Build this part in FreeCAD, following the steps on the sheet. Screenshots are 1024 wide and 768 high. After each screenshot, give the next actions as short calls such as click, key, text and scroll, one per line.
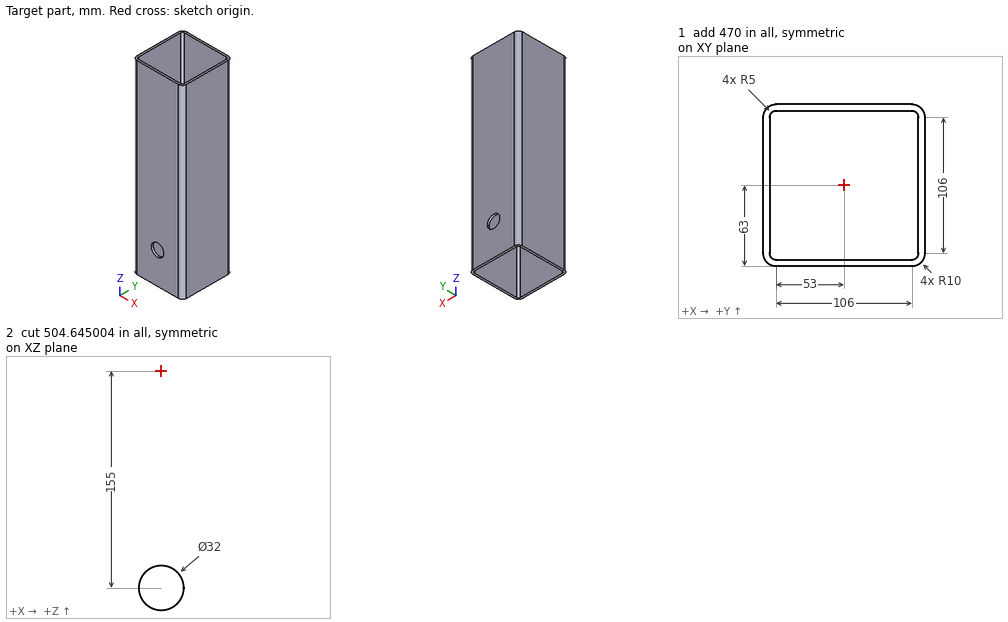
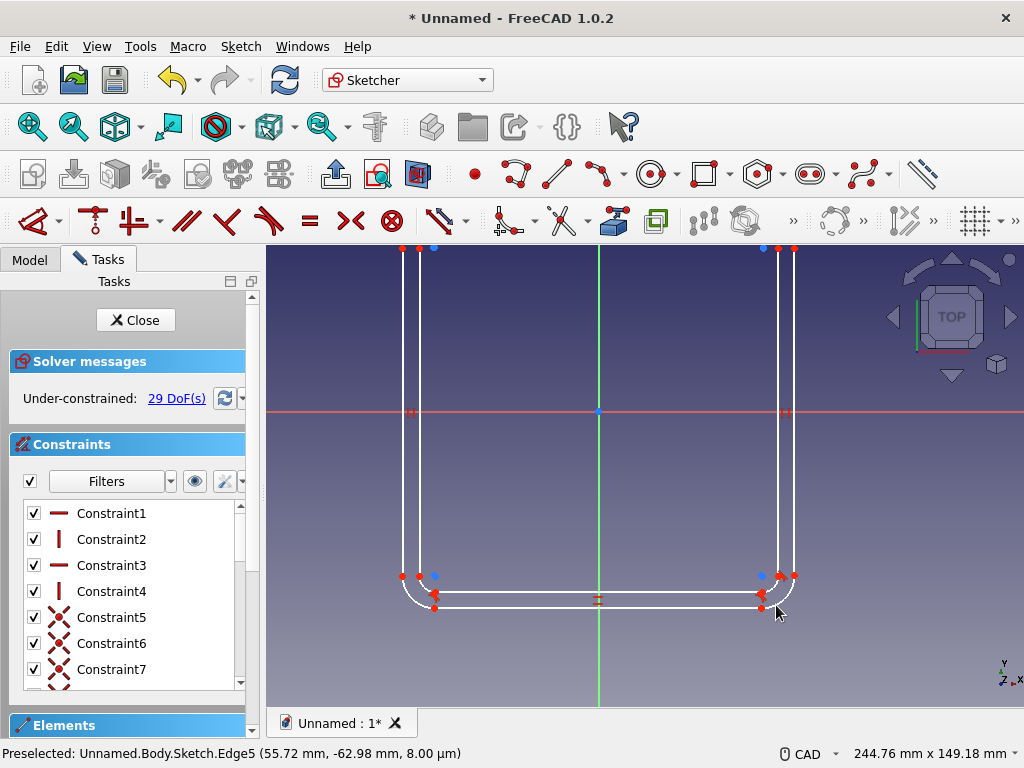
click(794, 477)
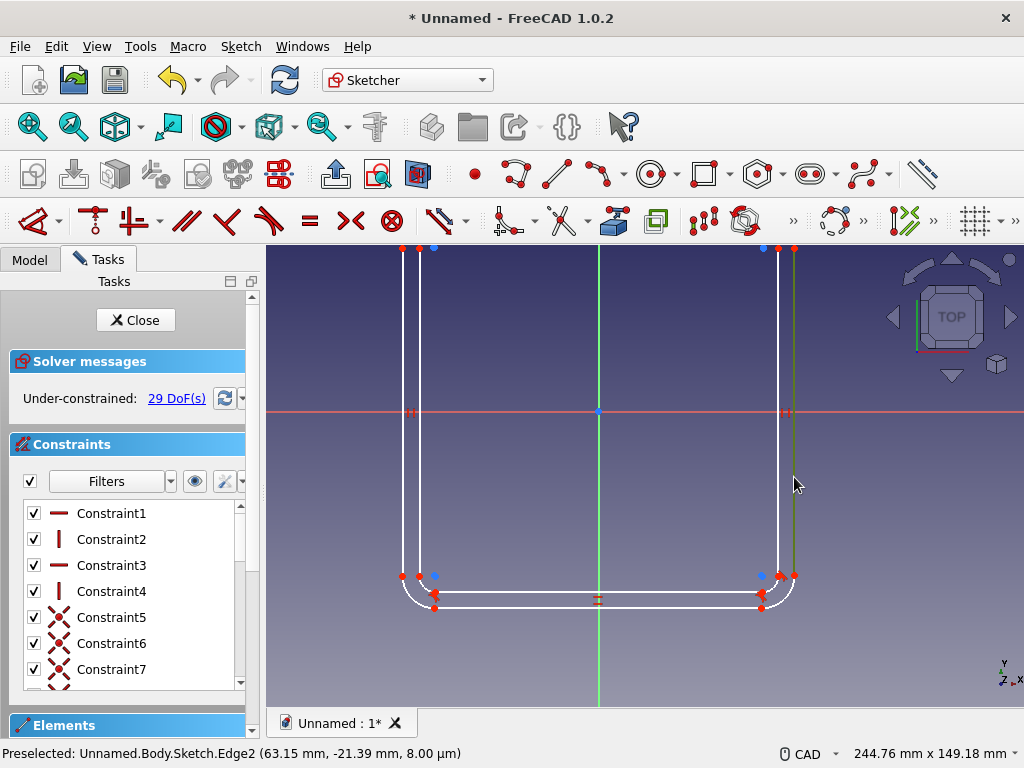
scroll(531, 607, down, 2)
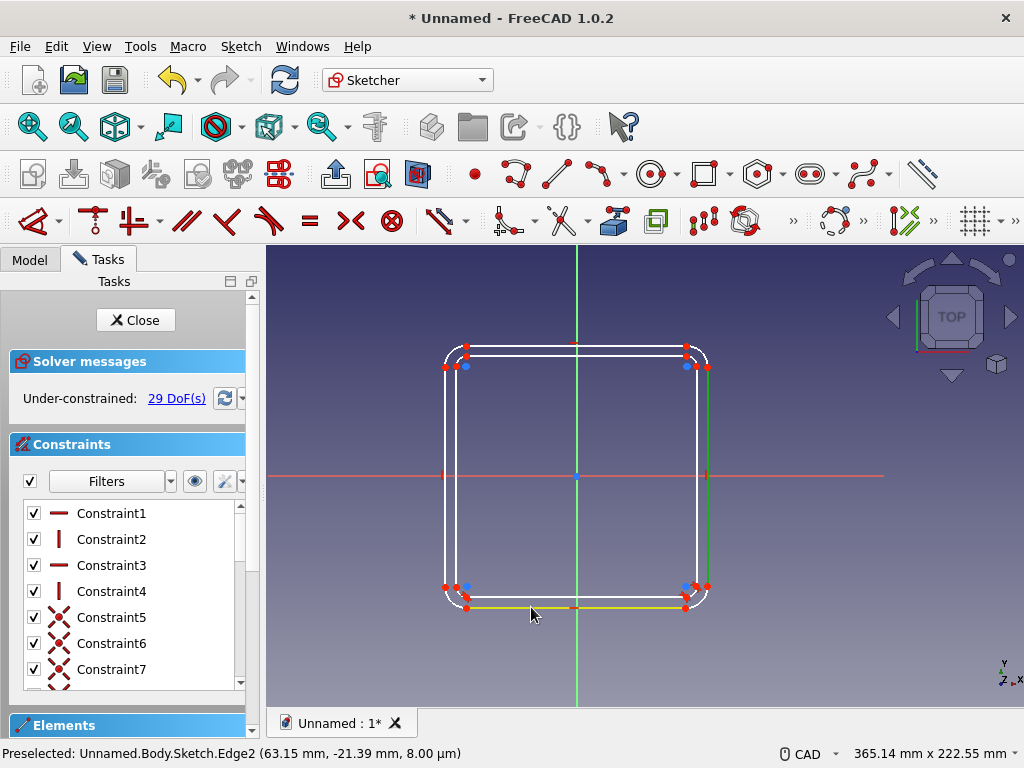
scroll(706, 358, up, 2)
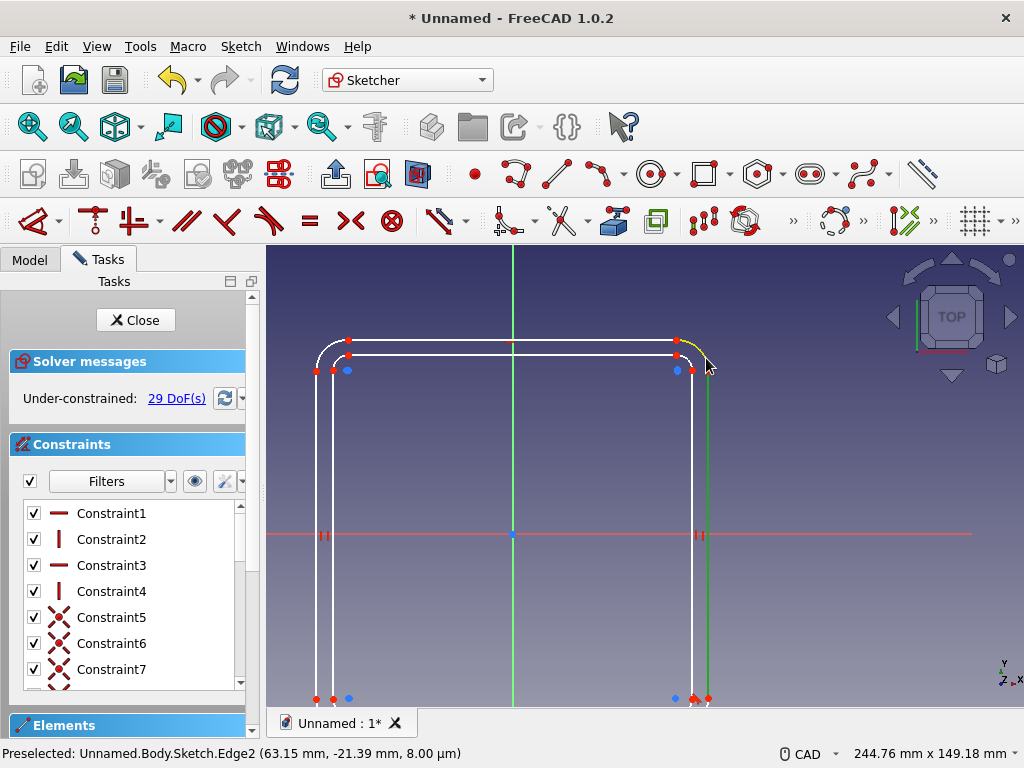
click(705, 357)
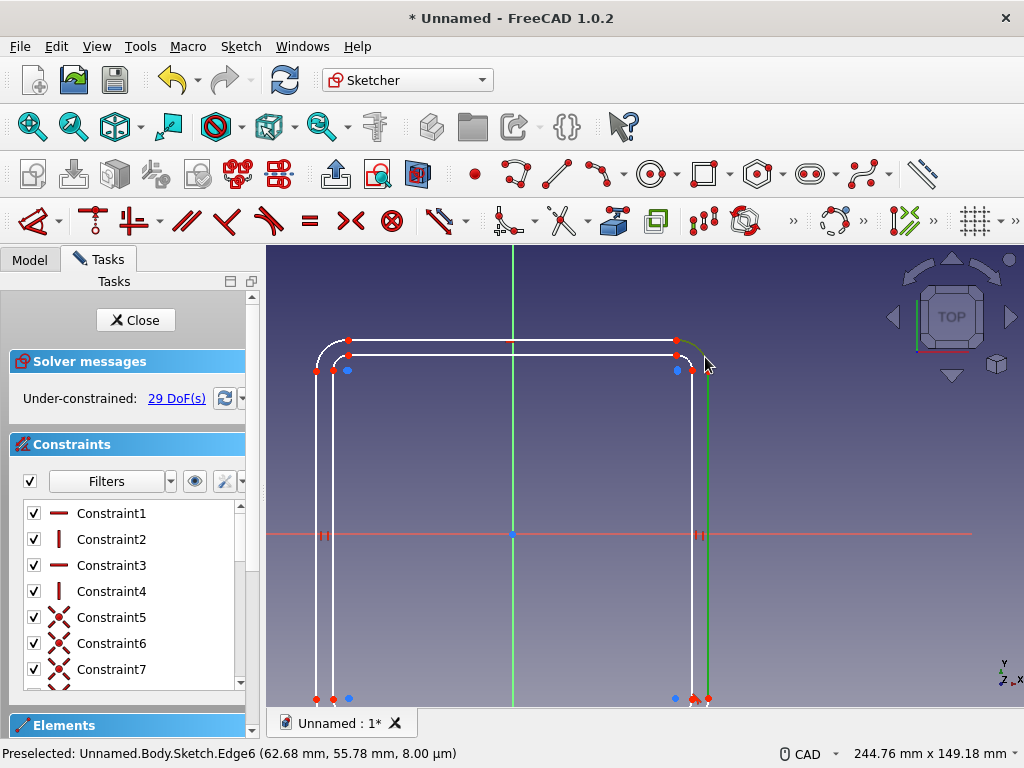
click(269, 222)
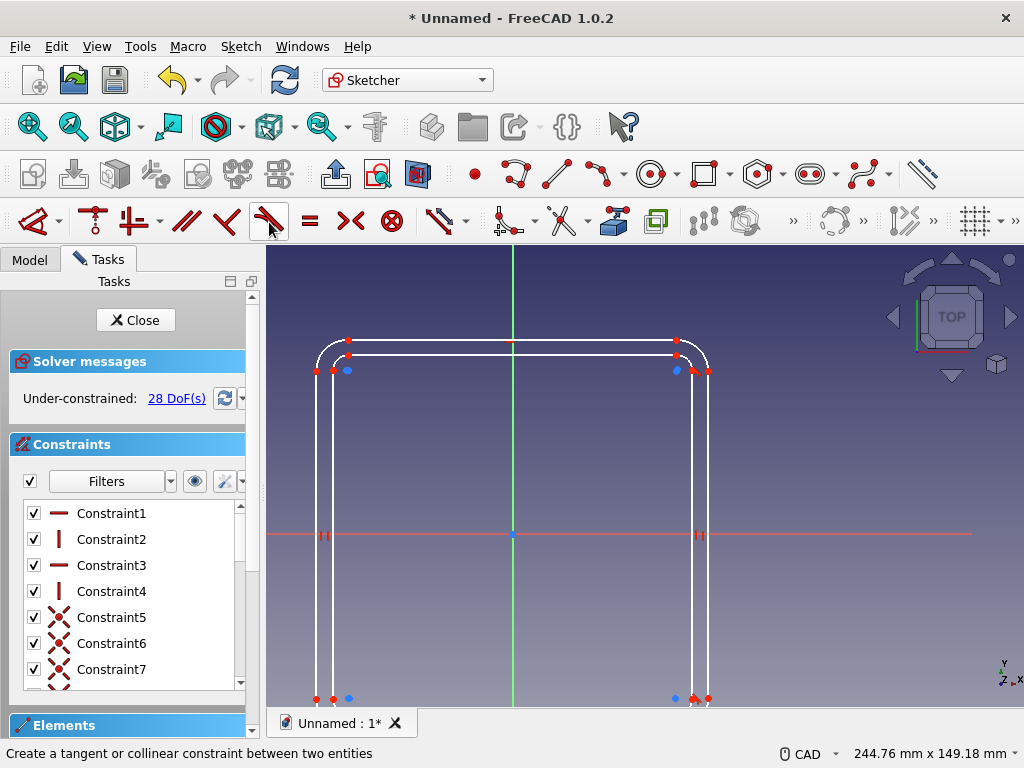
click(578, 340)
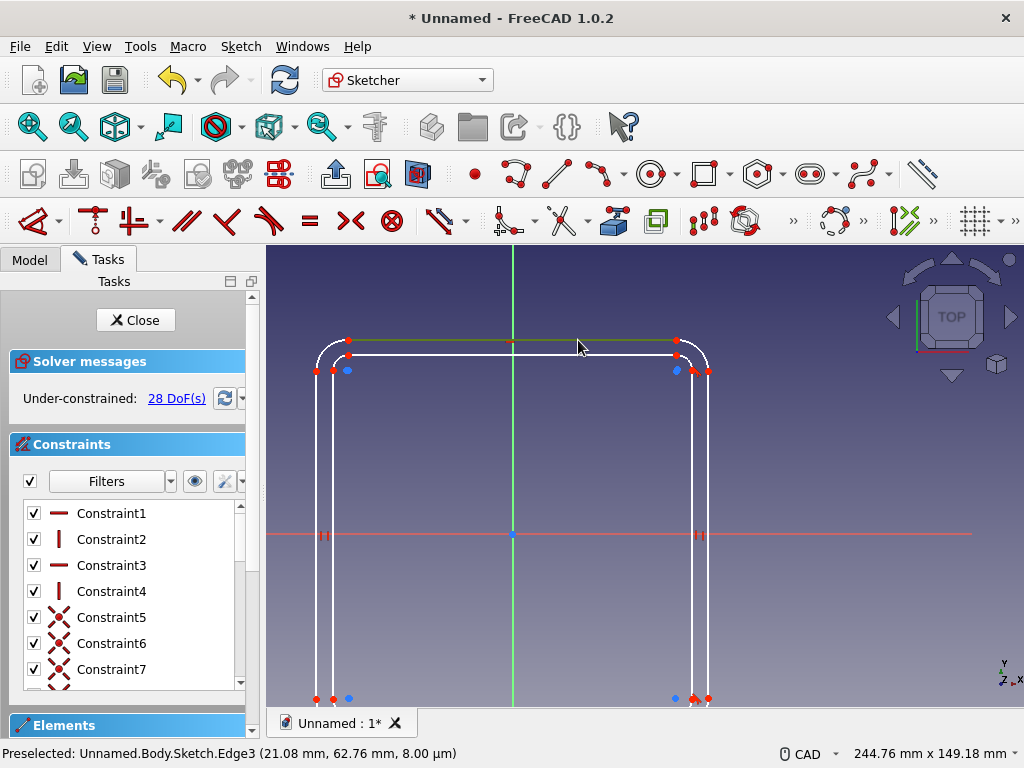
click(705, 357)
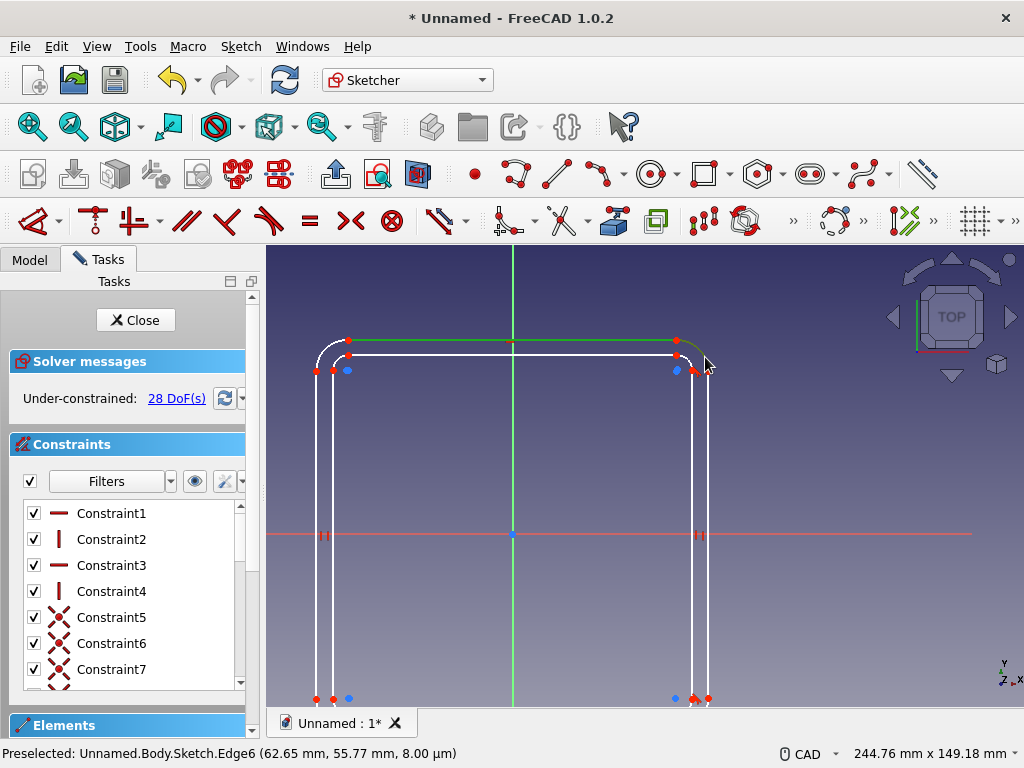
click(269, 222)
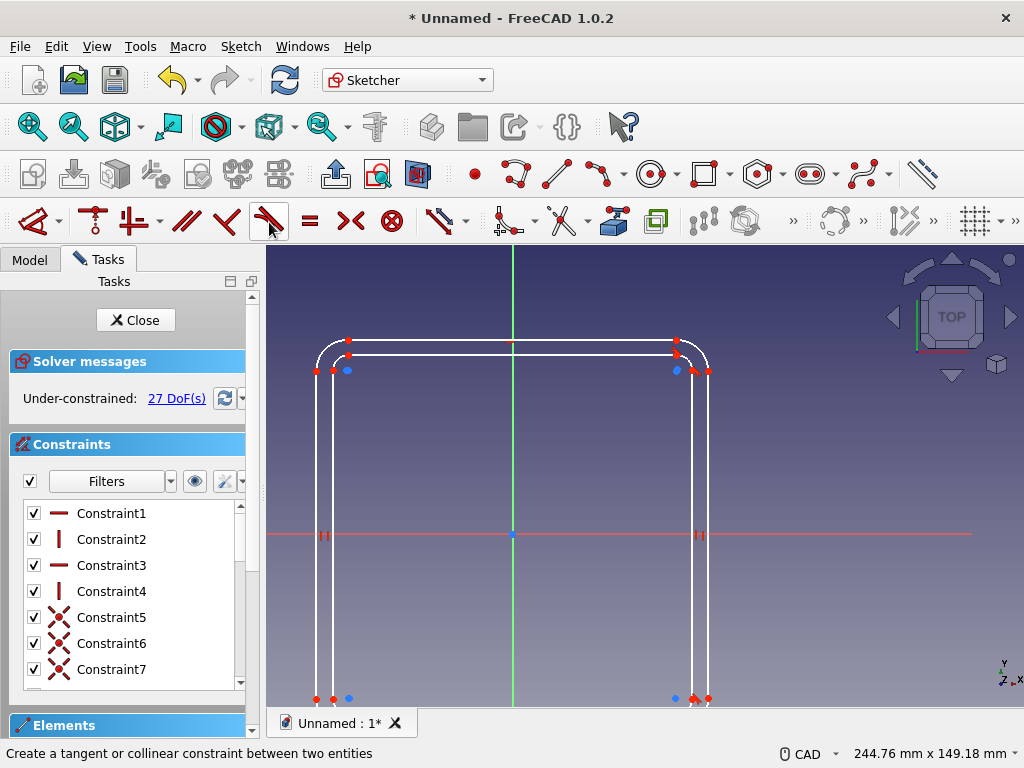
click(578, 340)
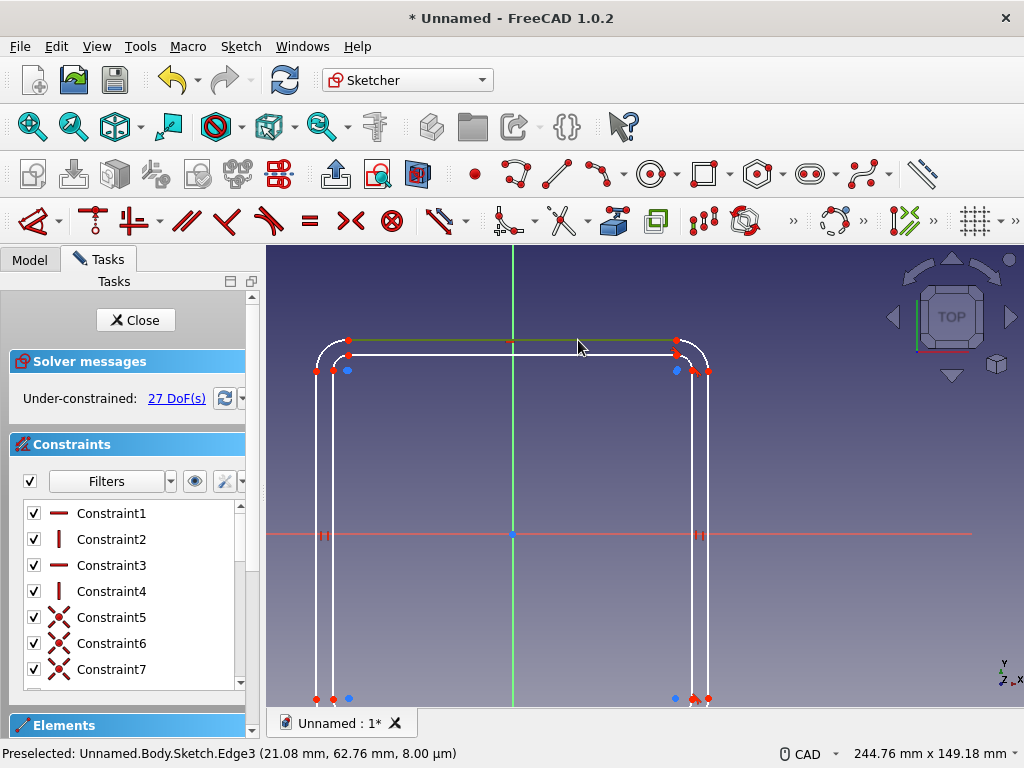
click(334, 343)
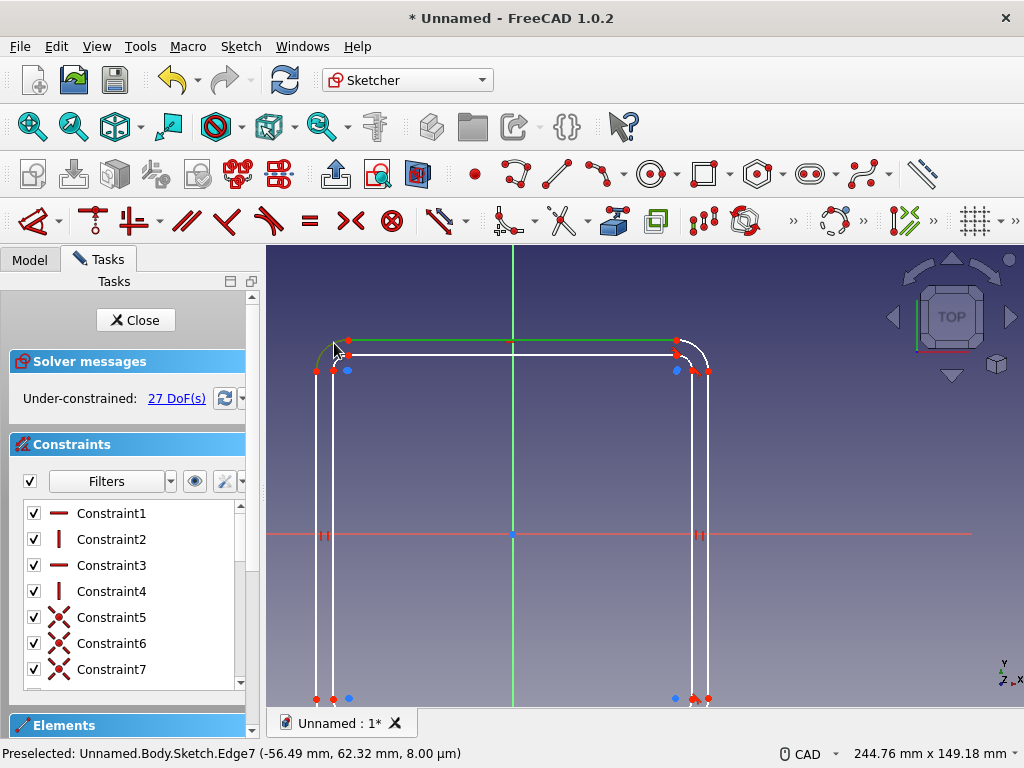
click(269, 222)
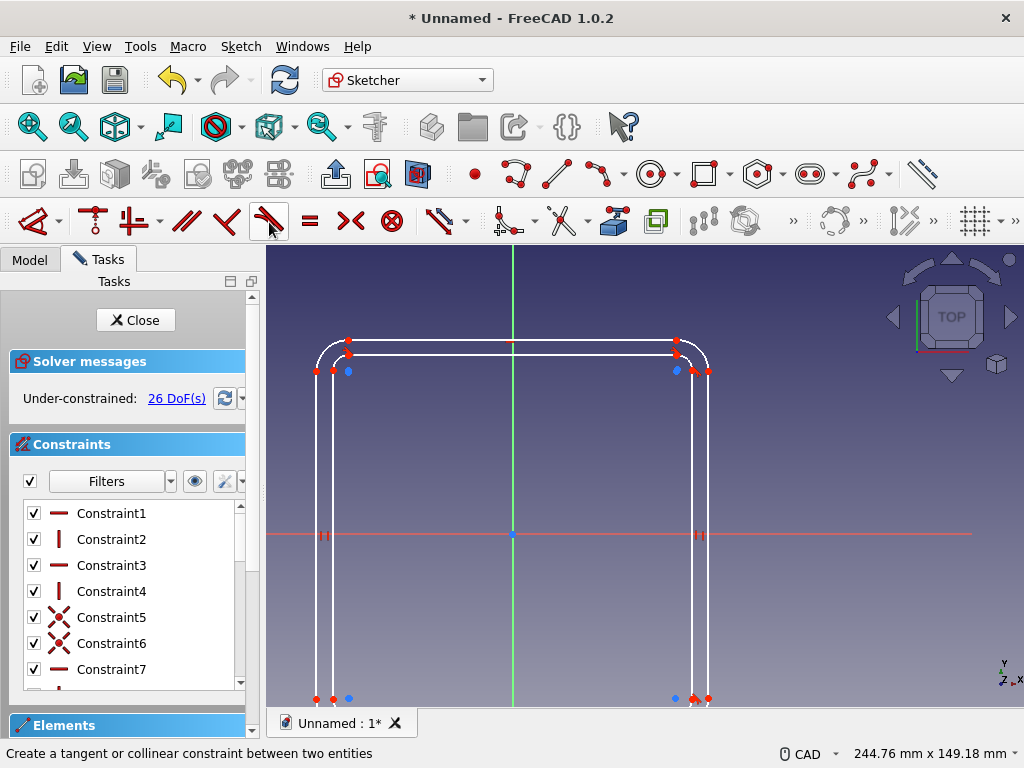
click(316, 470)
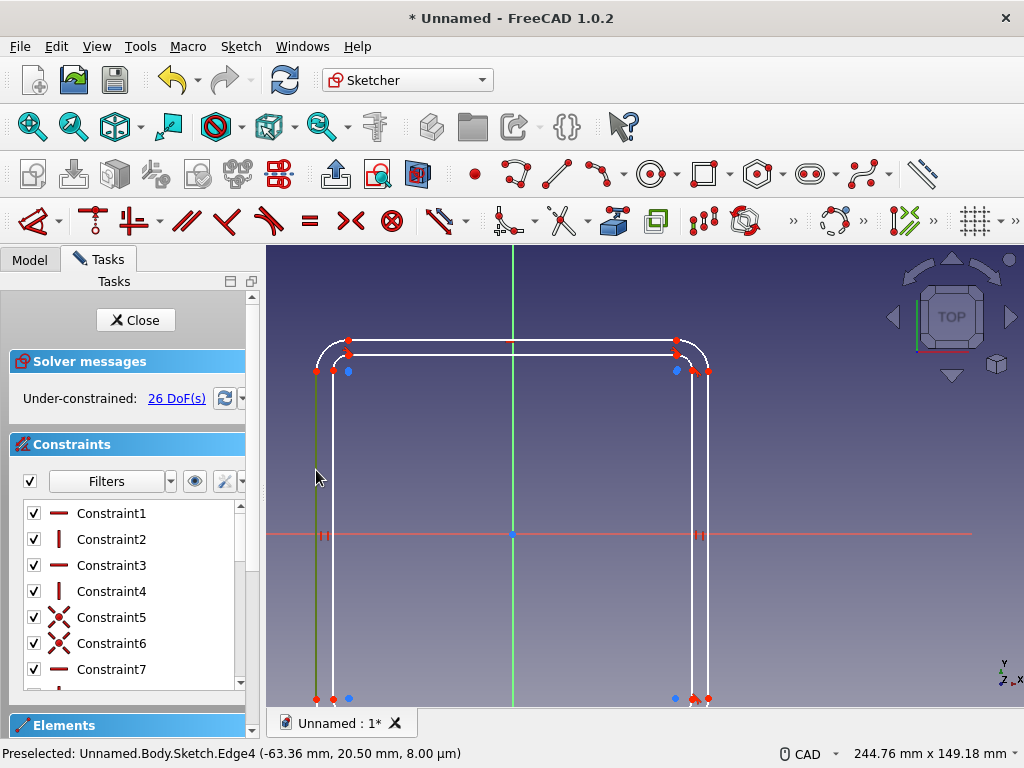
click(334, 343)